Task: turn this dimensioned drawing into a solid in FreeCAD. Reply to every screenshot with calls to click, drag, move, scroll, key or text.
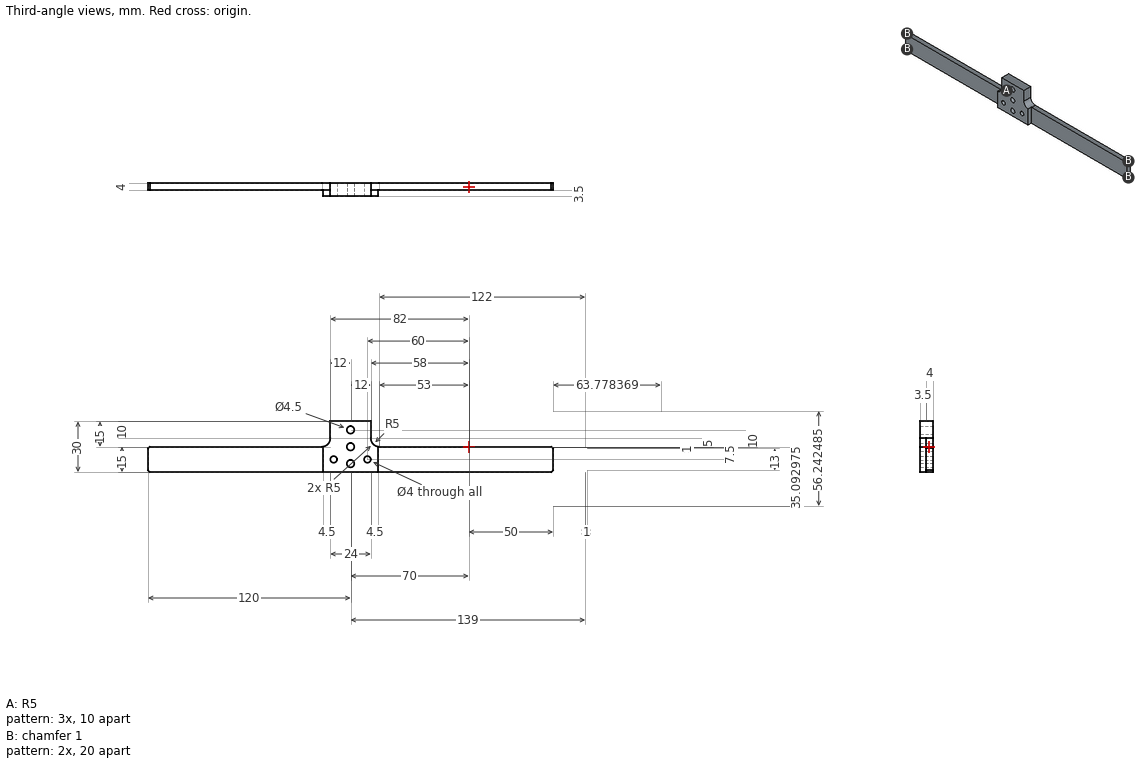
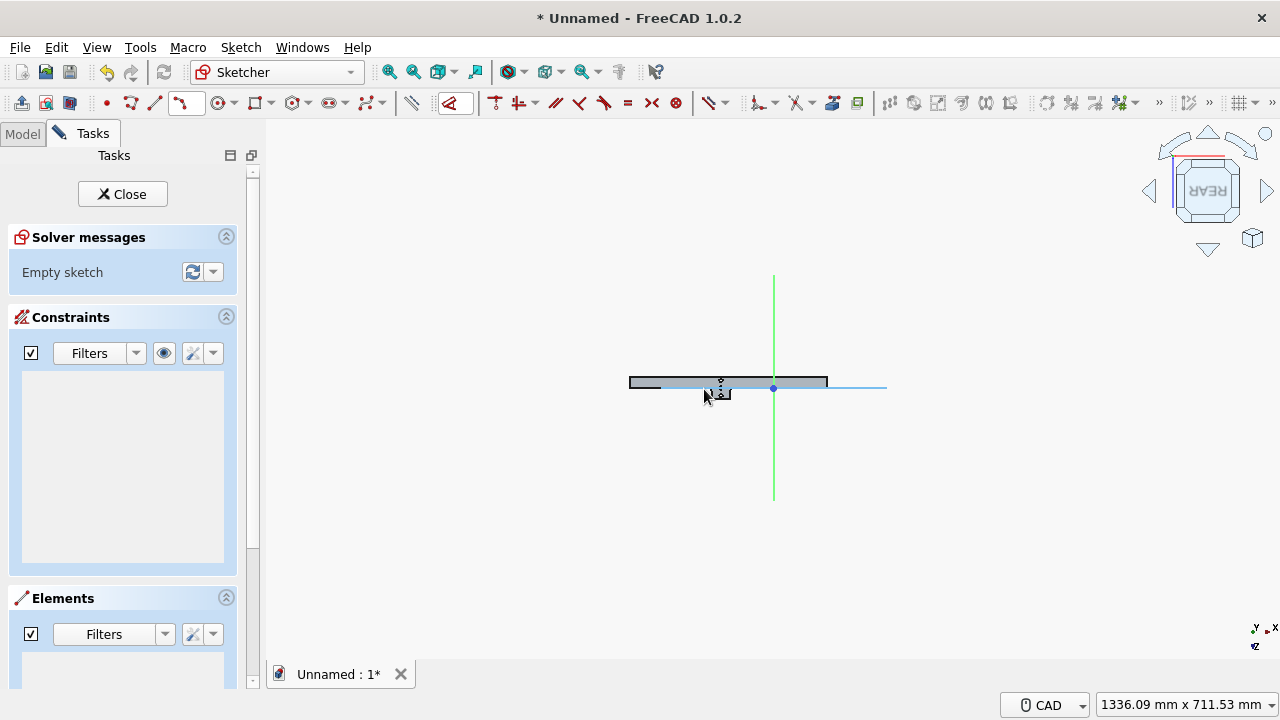
scroll(835, 382, up, 10)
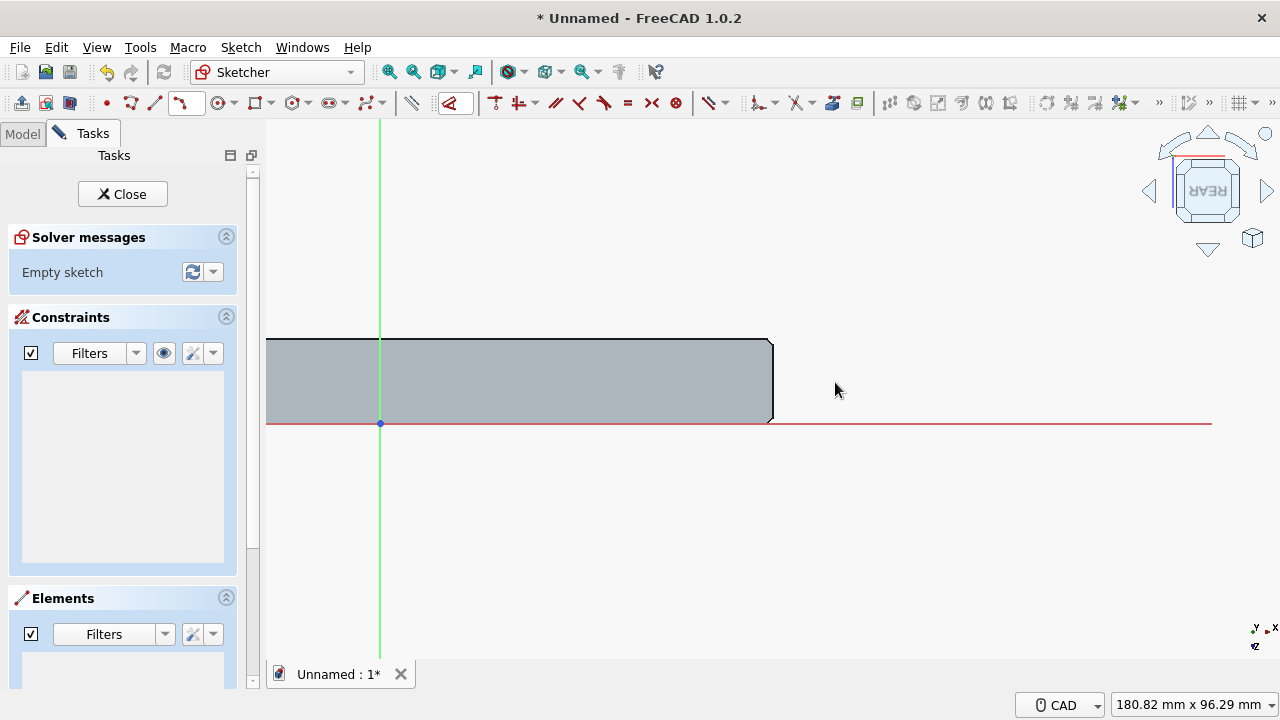
click(256, 104)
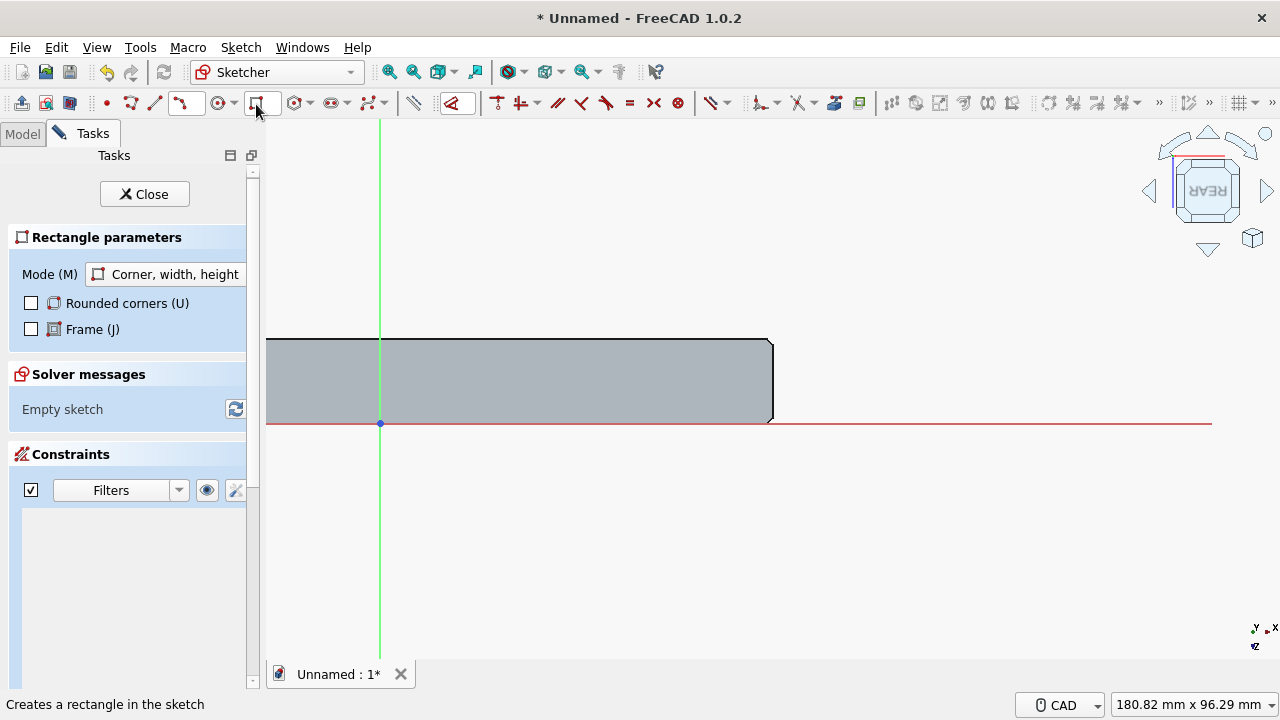
click(661, 227)
click(1018, 542)
key(Escape)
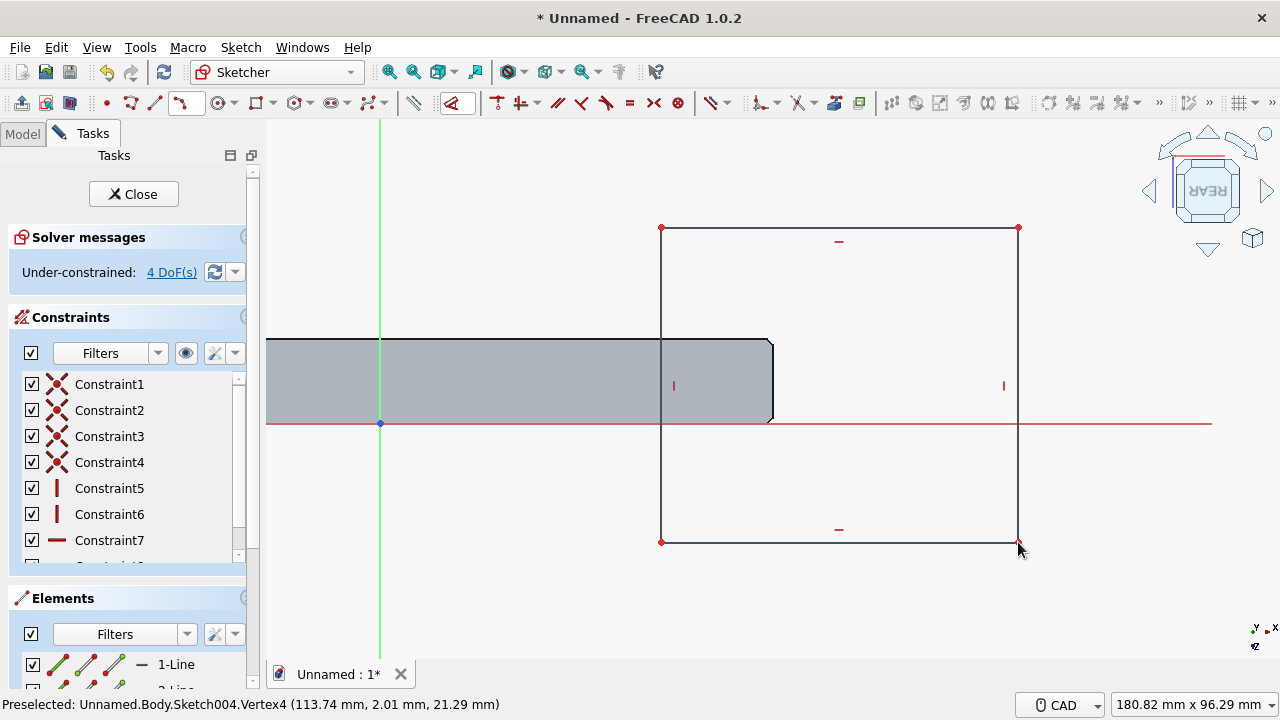
click(661, 228)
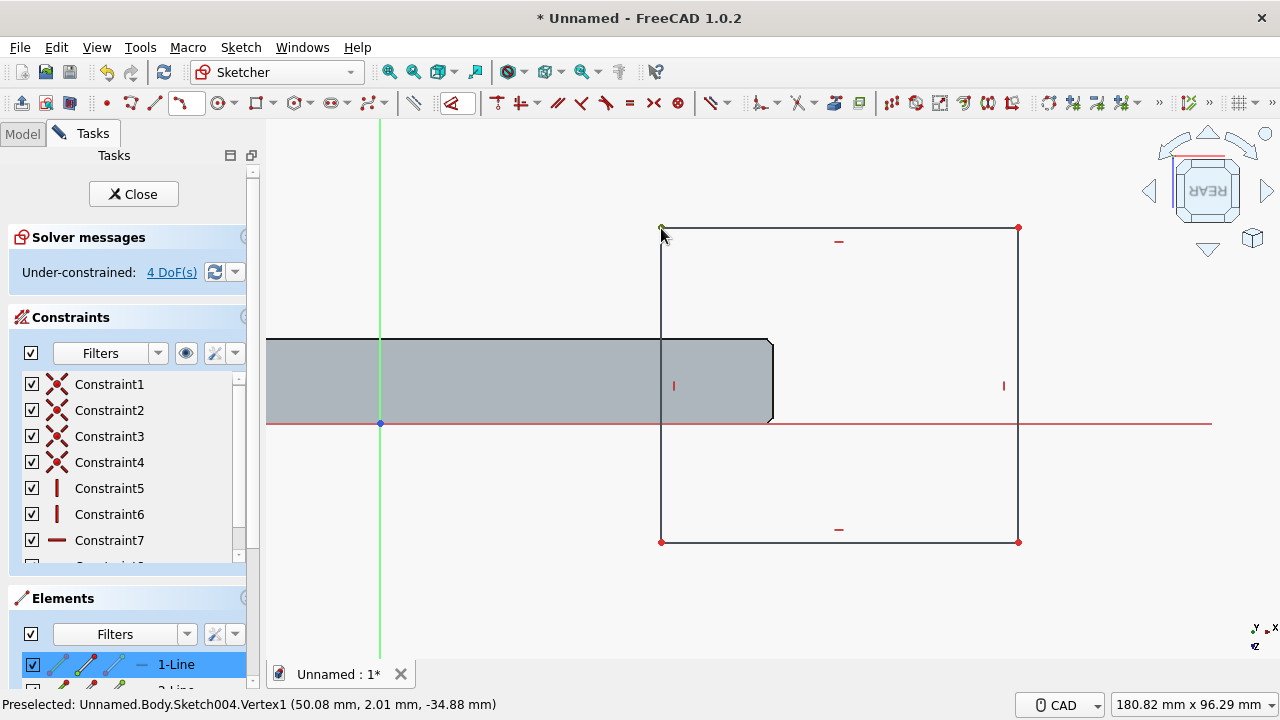
key(l)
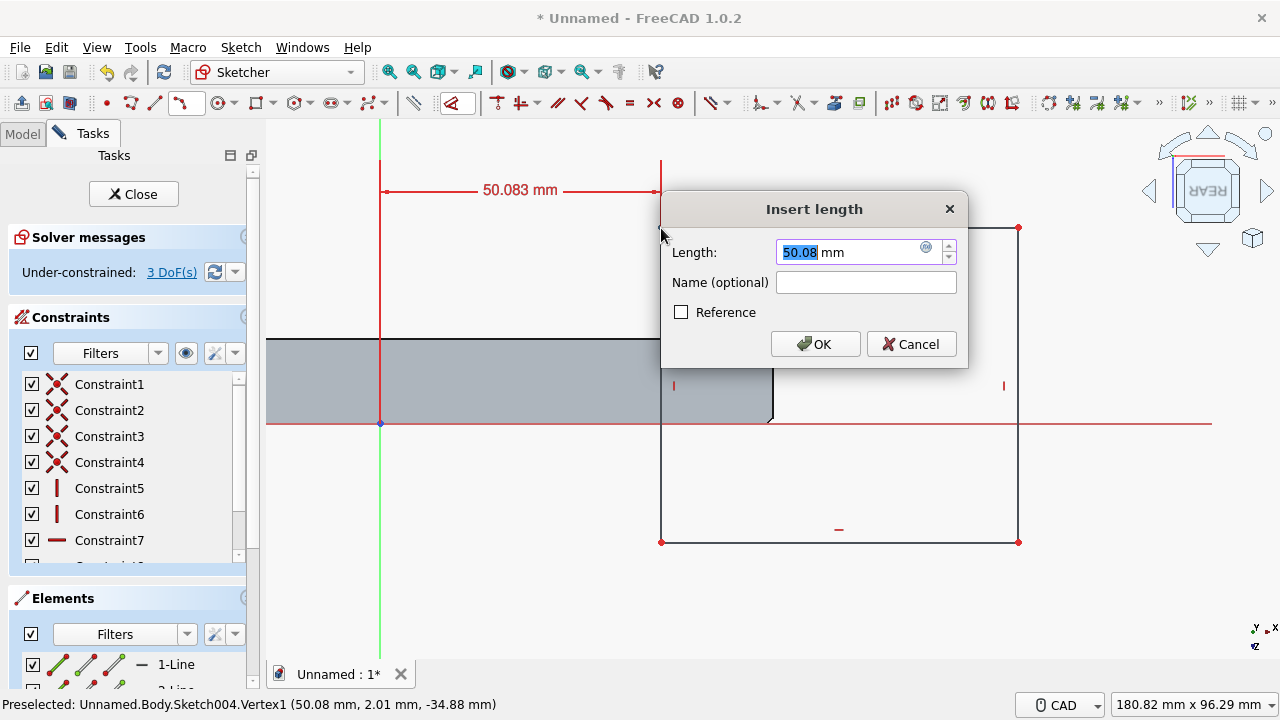
text(50)
key(Return)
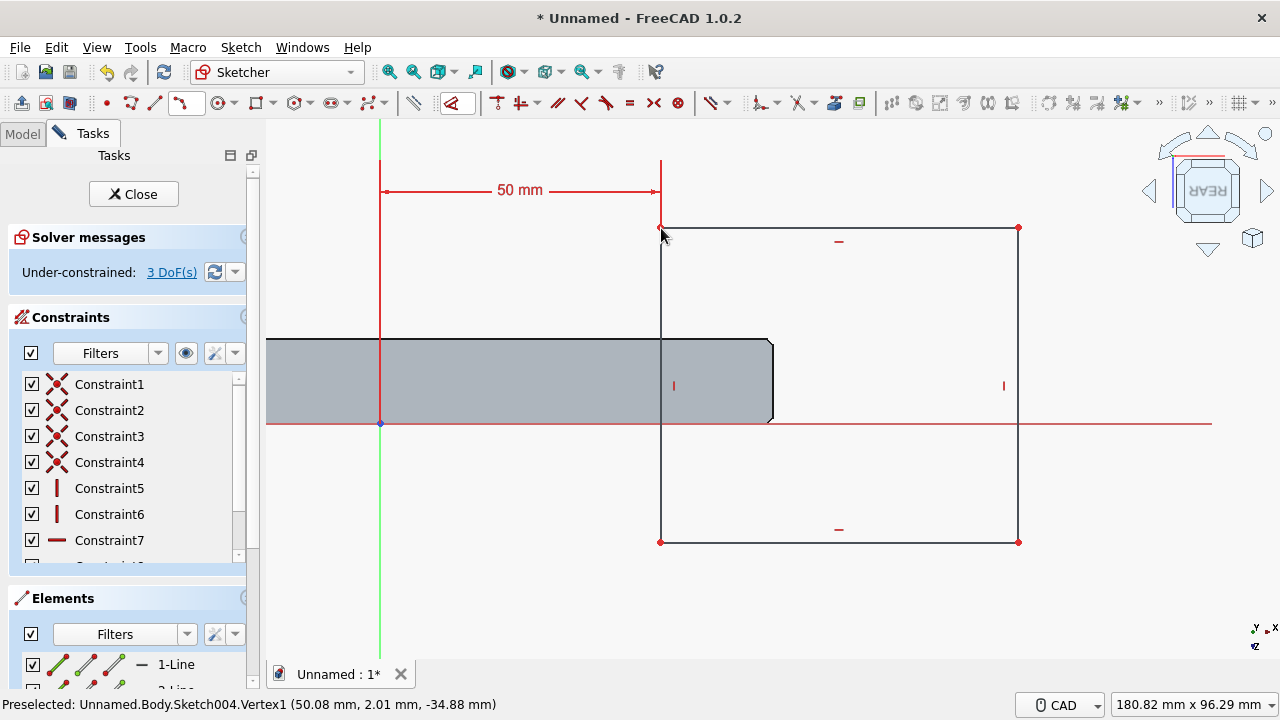
click(661, 322)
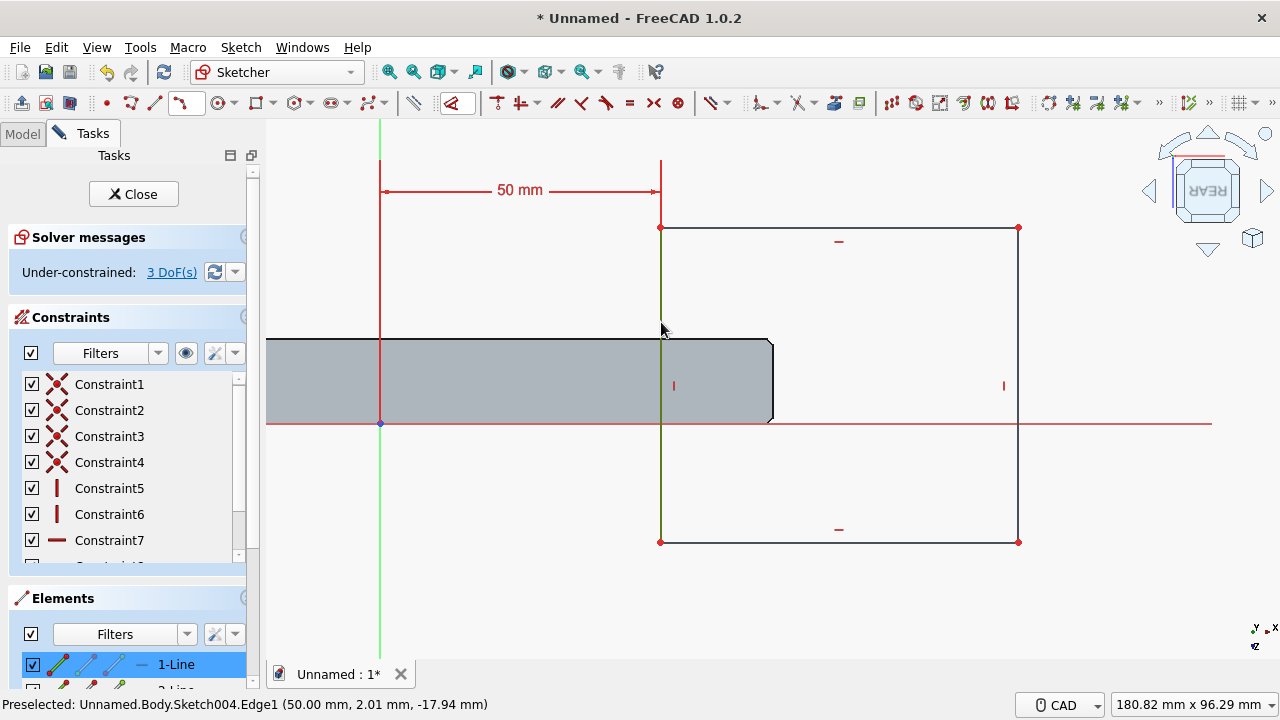
click(470, 104)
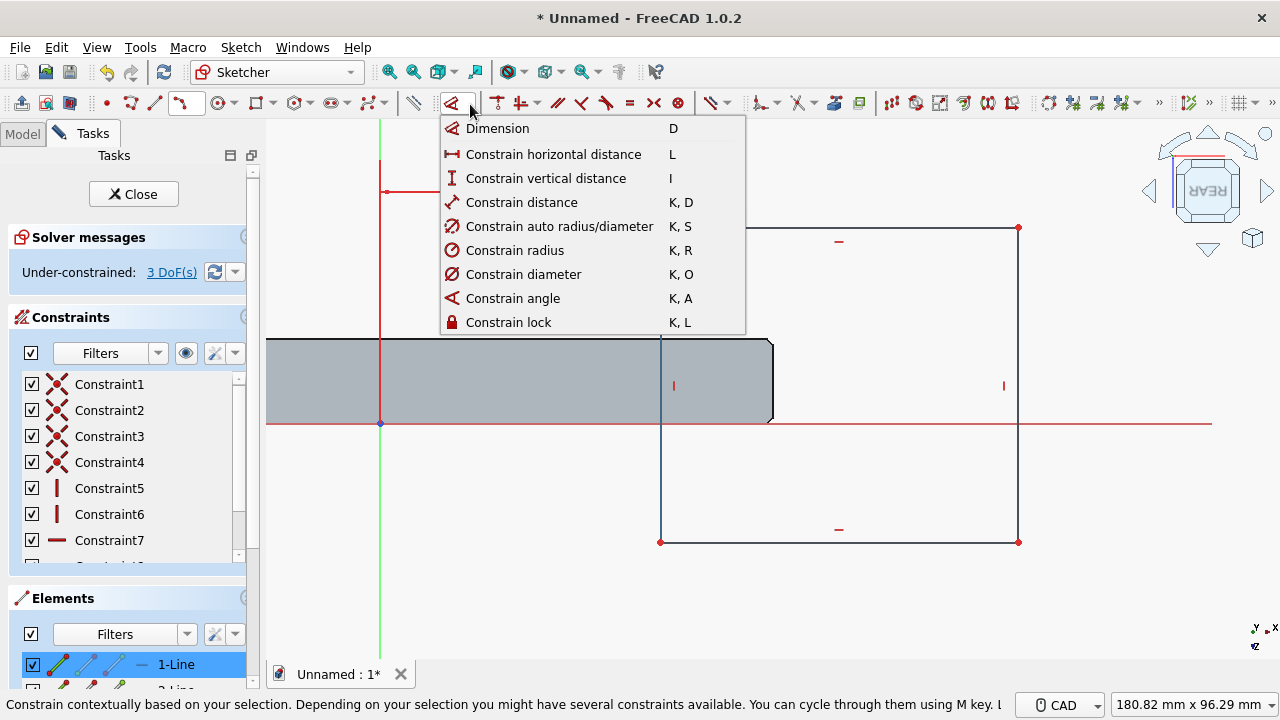
click(593, 178)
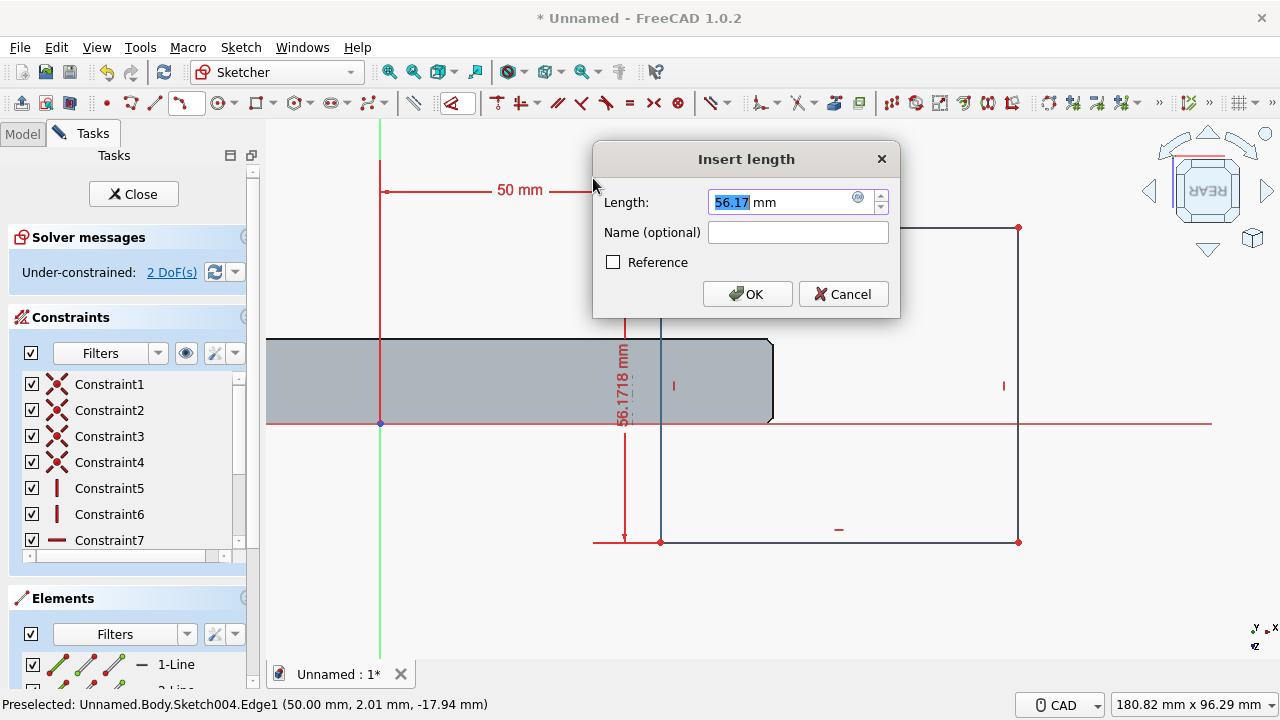
text(56.242485)
key(Return)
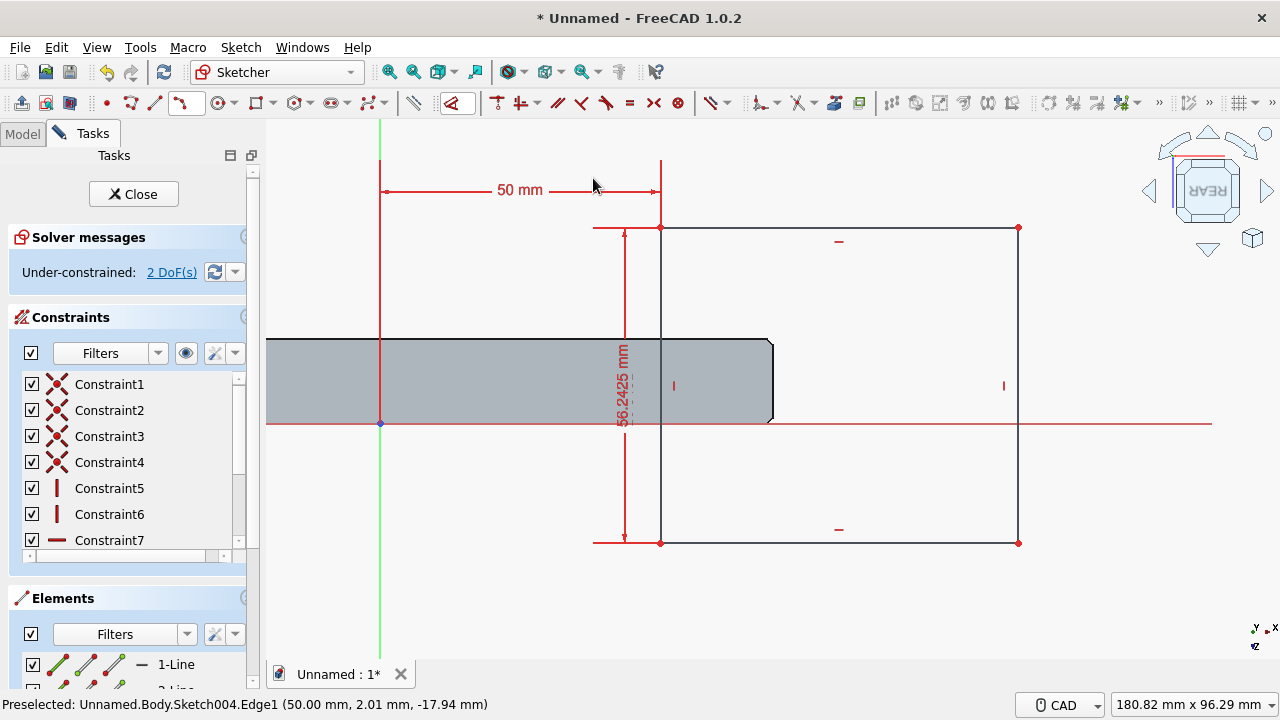
click(768, 543)